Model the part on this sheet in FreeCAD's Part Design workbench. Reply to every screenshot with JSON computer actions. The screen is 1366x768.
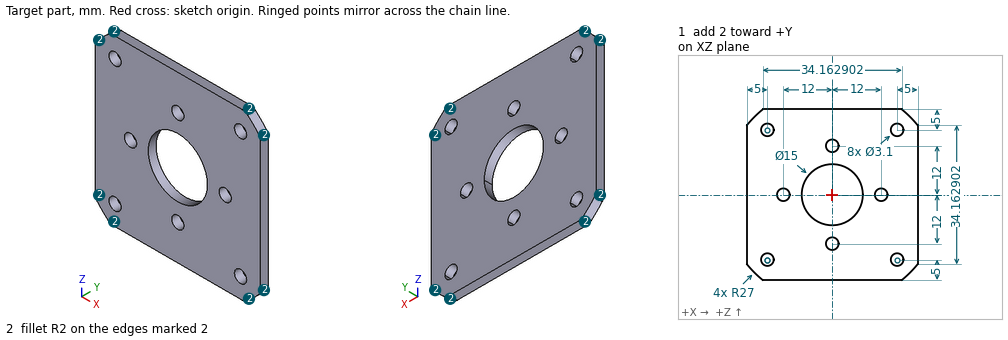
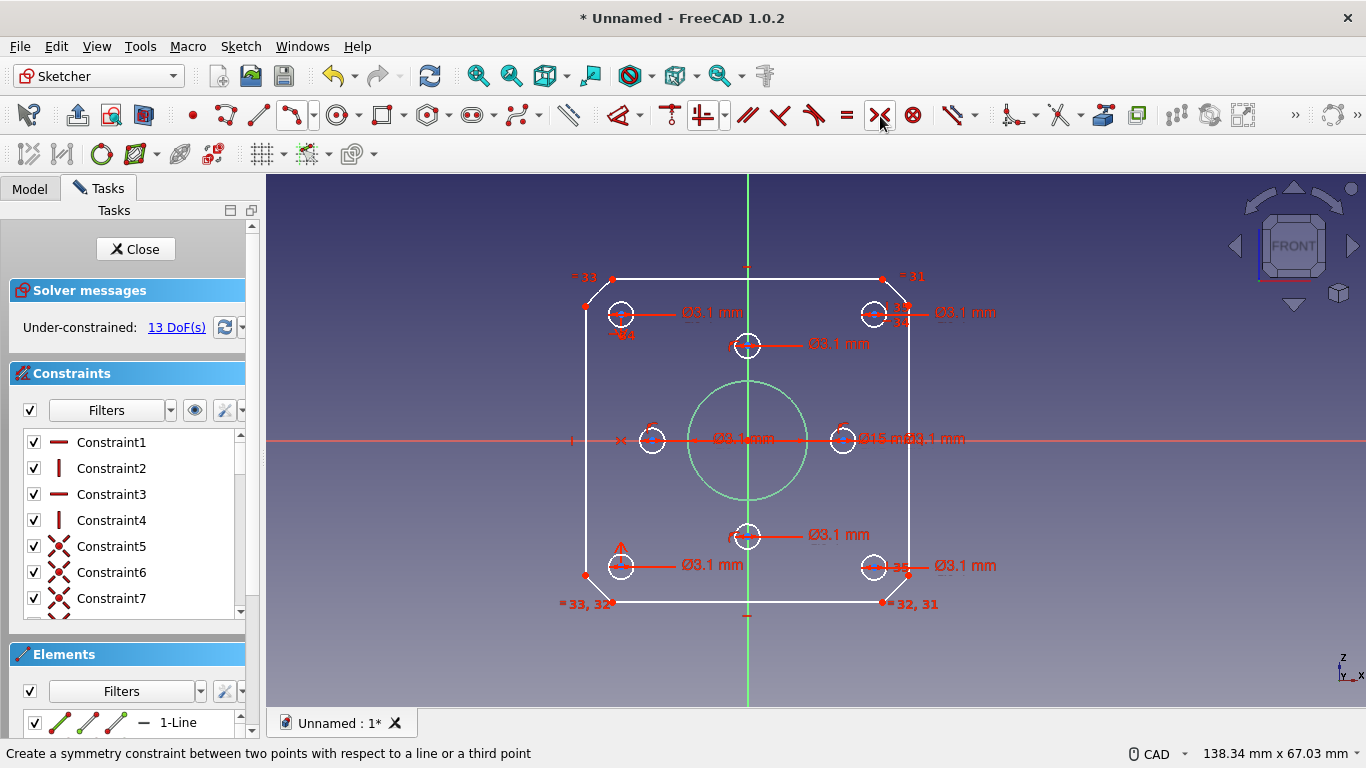
{"action": "left_click", "coordinate": [874, 568]}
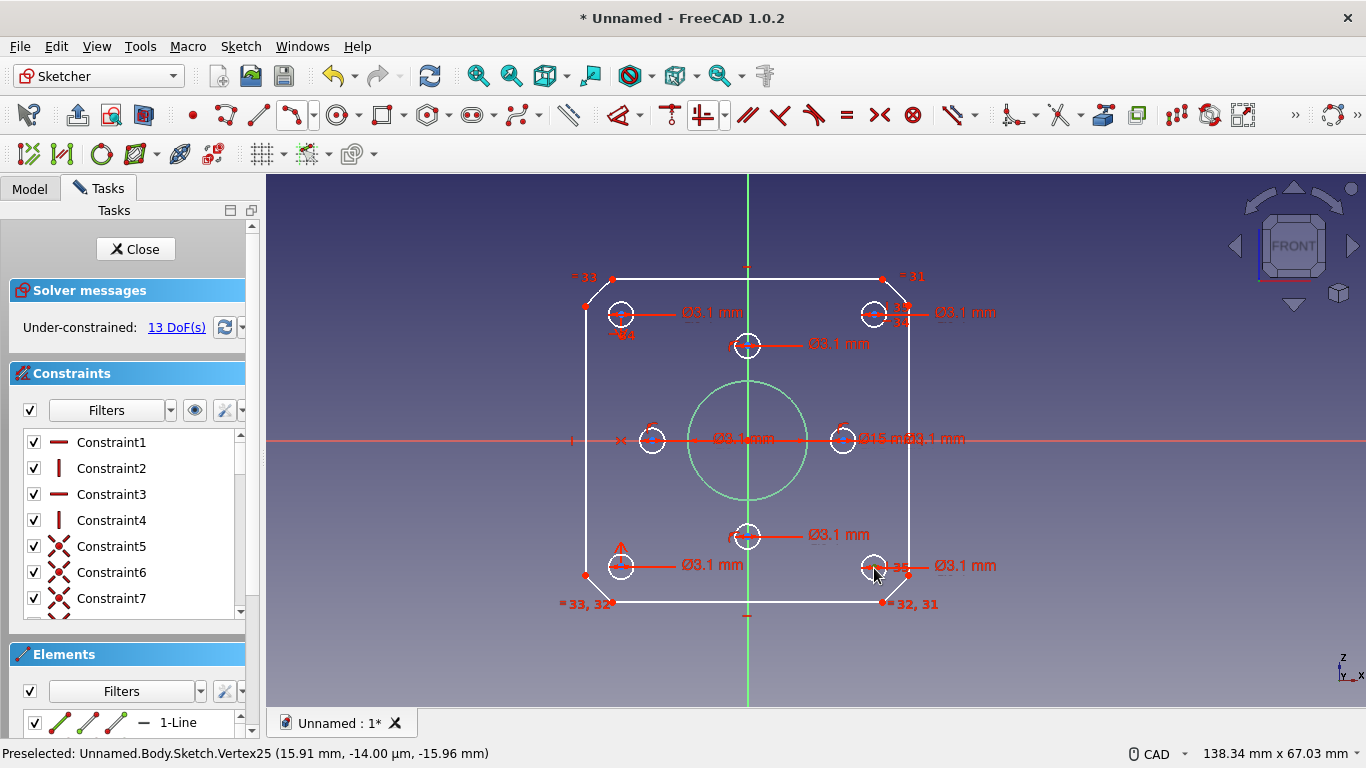
{"action": "left_click", "coordinate": [621, 567]}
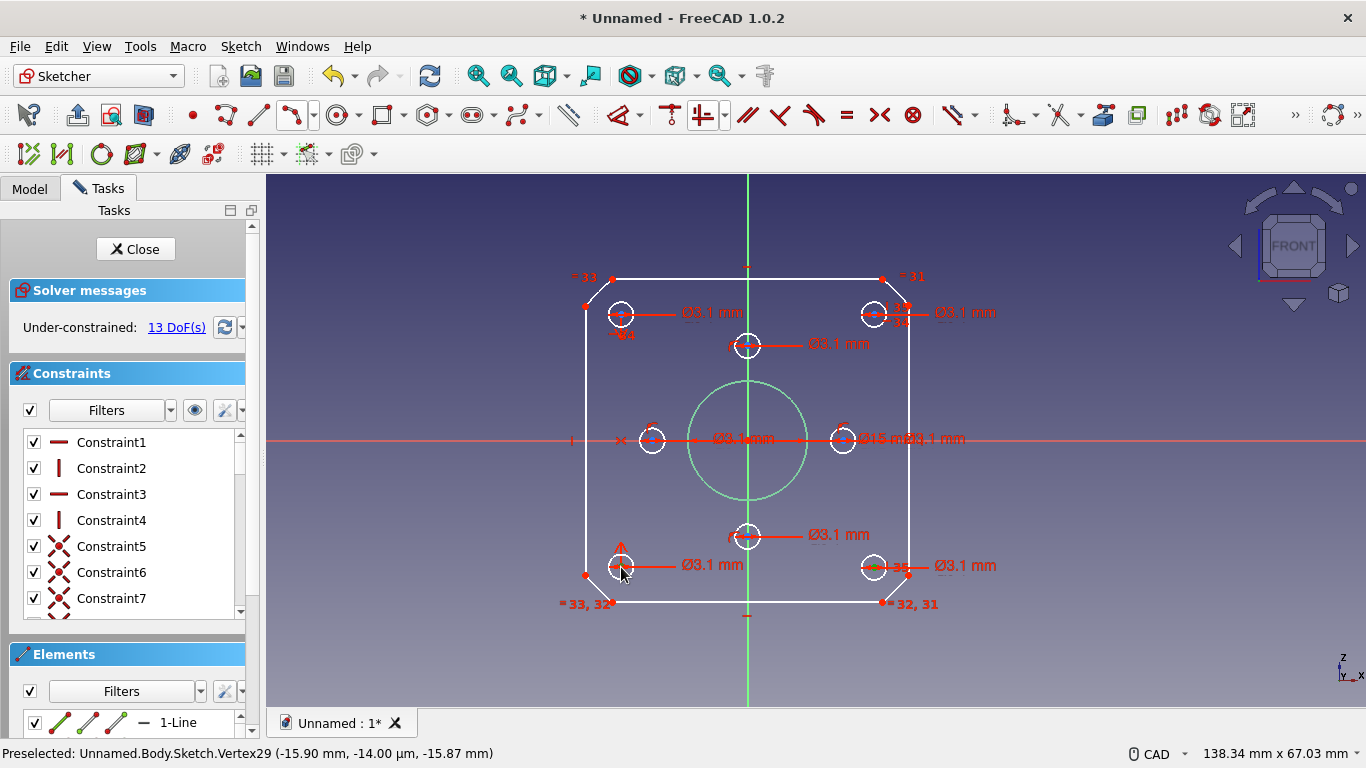
{"action": "left_click", "coordinate": [748, 645]}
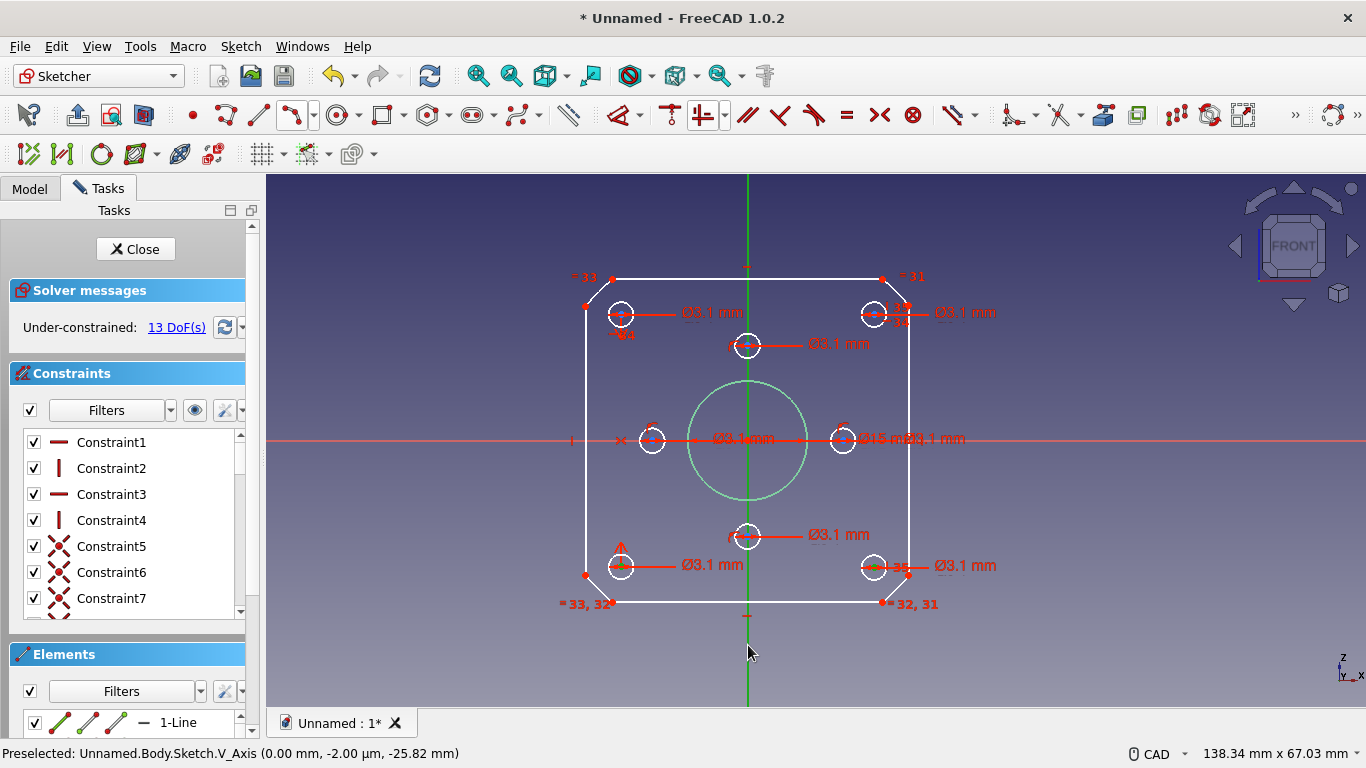
{"action": "left_click", "coordinate": [880, 116]}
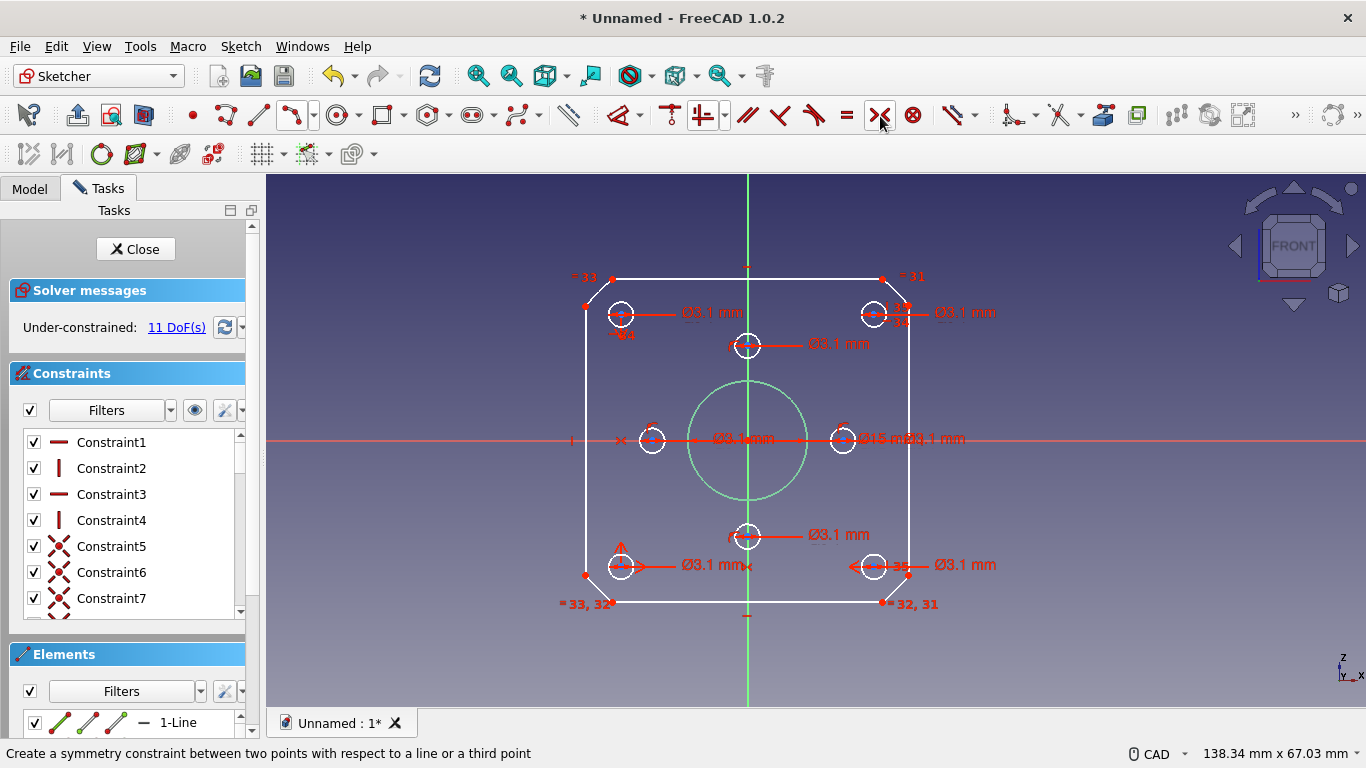
{"action": "left_click", "coordinate": [618, 116]}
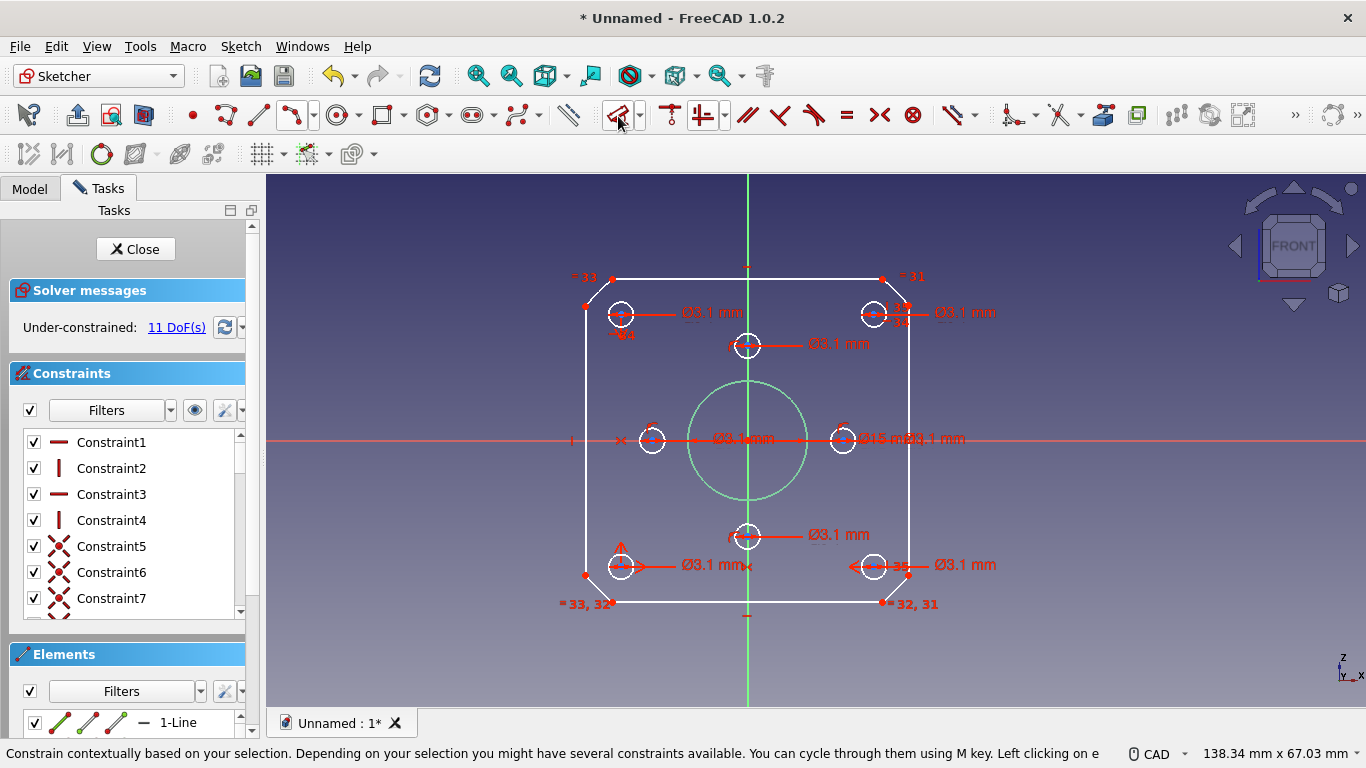
{"action": "scroll", "coordinate": [902, 297], "scroll_direction": "up", "scroll_amount": 2}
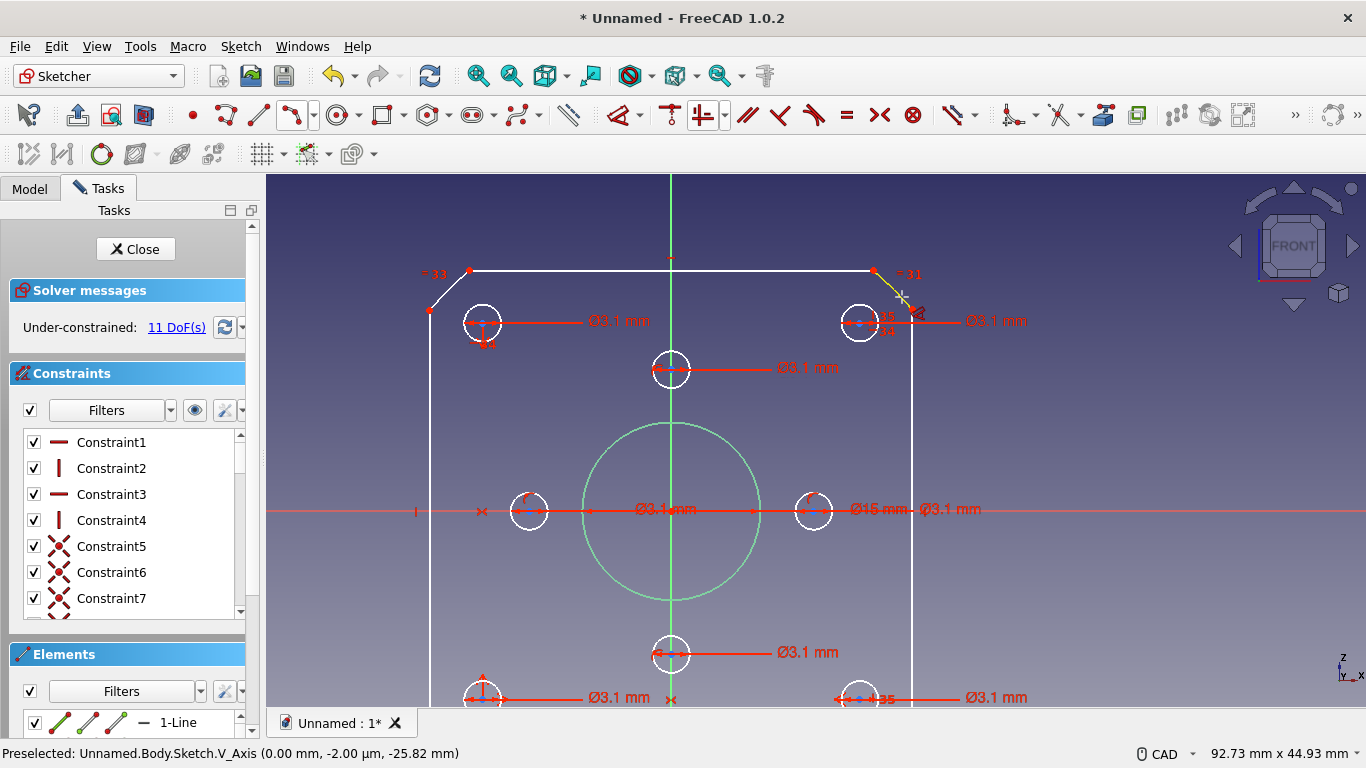
{"action": "left_click", "coordinate": [901, 297]}
{"action": "left_click", "coordinate": [924, 275]}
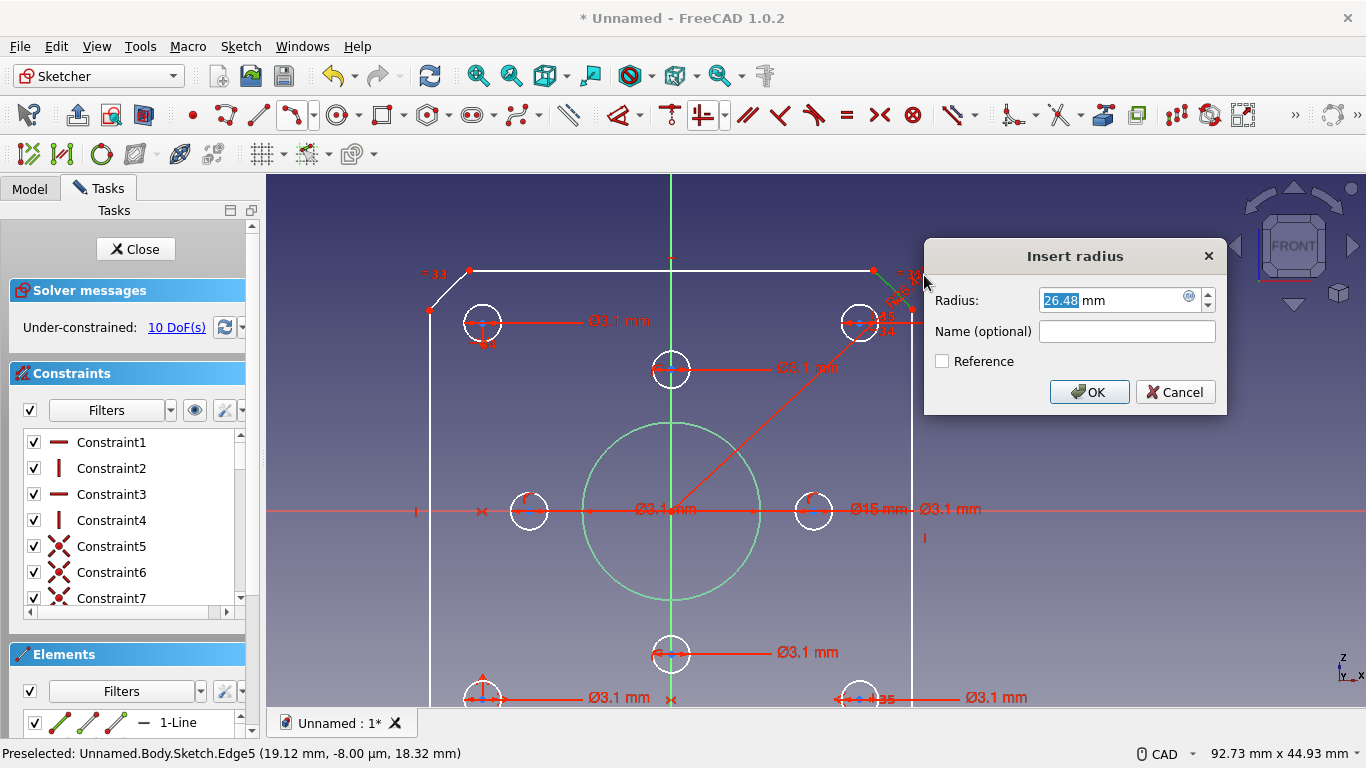
{"action": "type", "text": "27"}
{"action": "key", "text": "Return"}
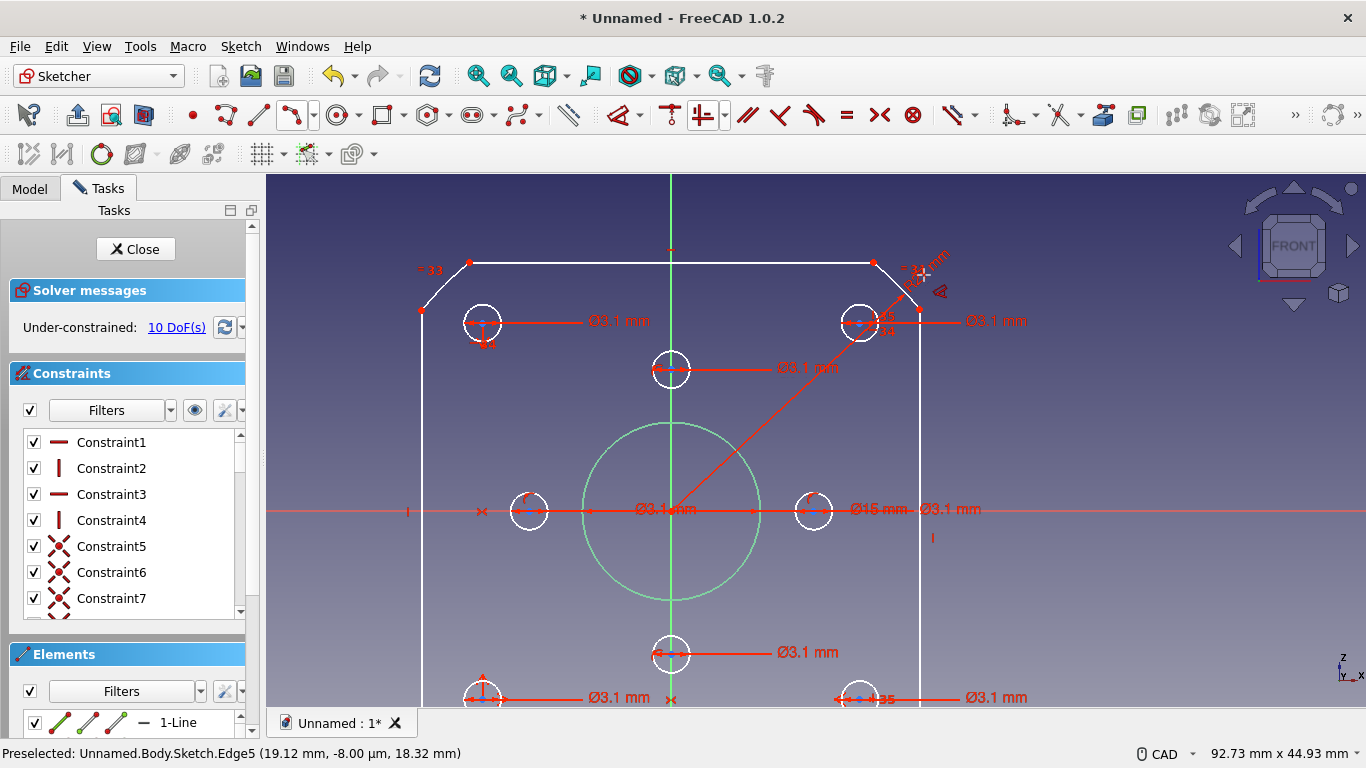
{"action": "left_click", "coordinate": [671, 370]}
{"action": "left_click", "coordinate": [705, 408]}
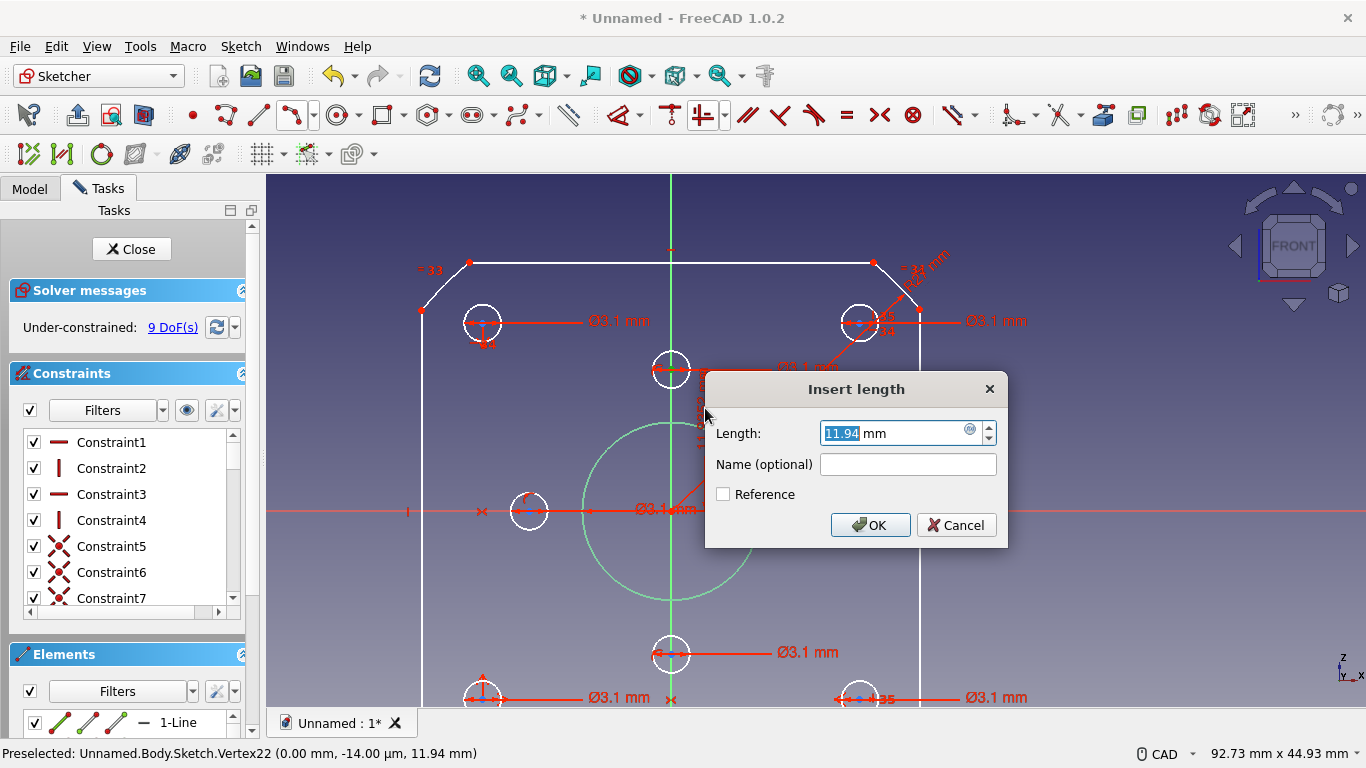
{"action": "type", "text": "12"}
{"action": "key", "text": "Return"}